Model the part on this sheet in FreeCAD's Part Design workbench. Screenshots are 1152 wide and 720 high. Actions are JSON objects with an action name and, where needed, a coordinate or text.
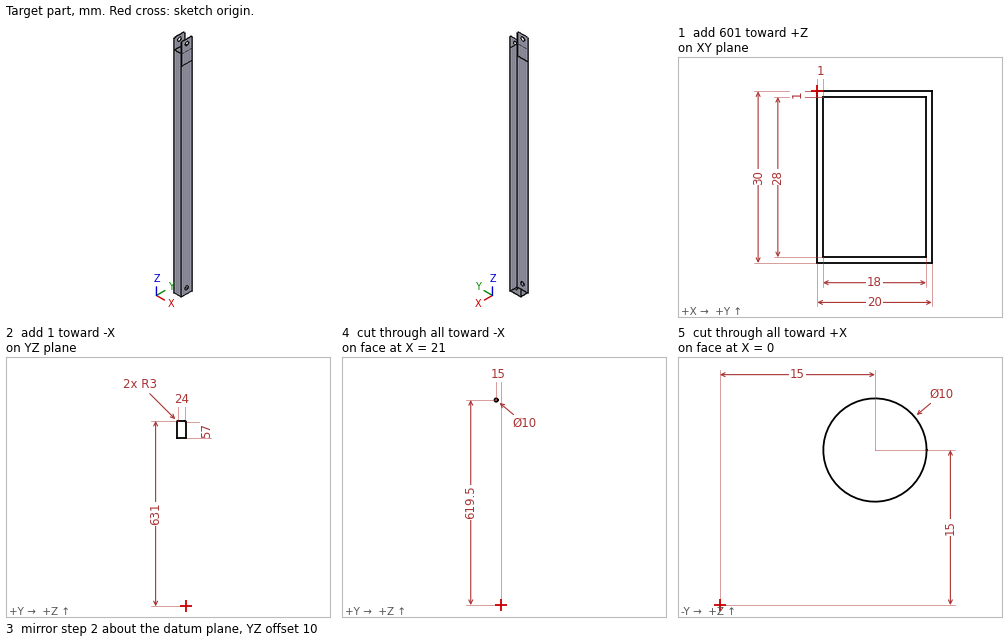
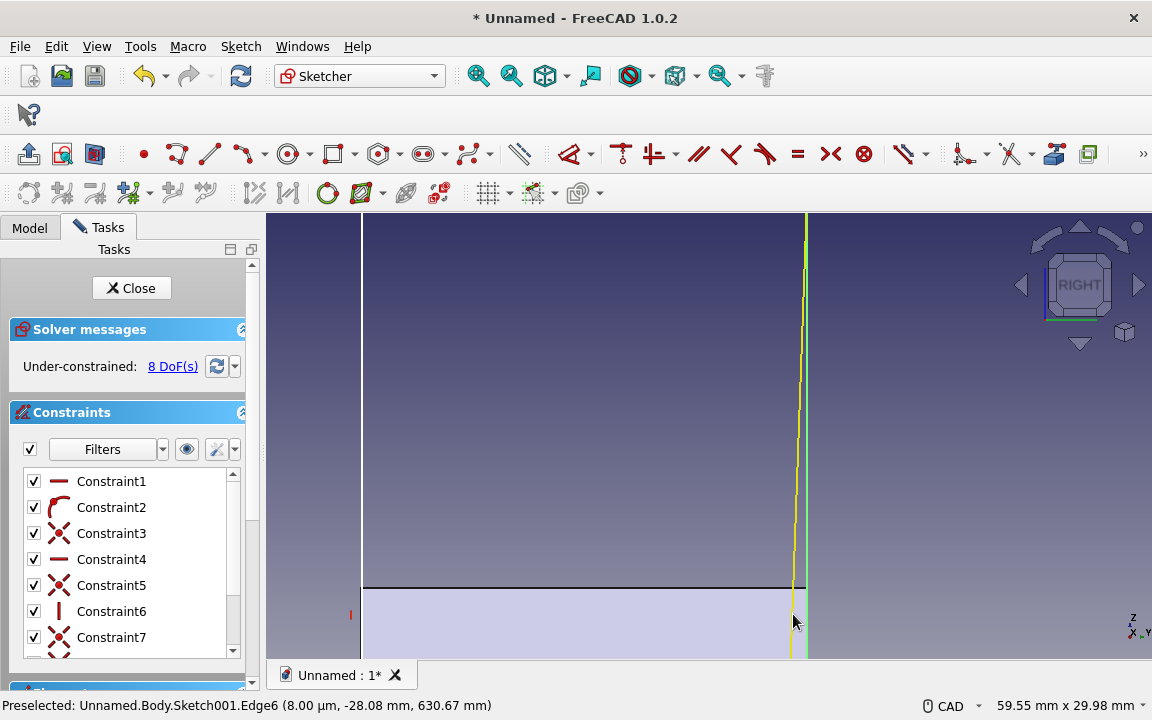
{"action": "left_click", "coordinate": [792, 614]}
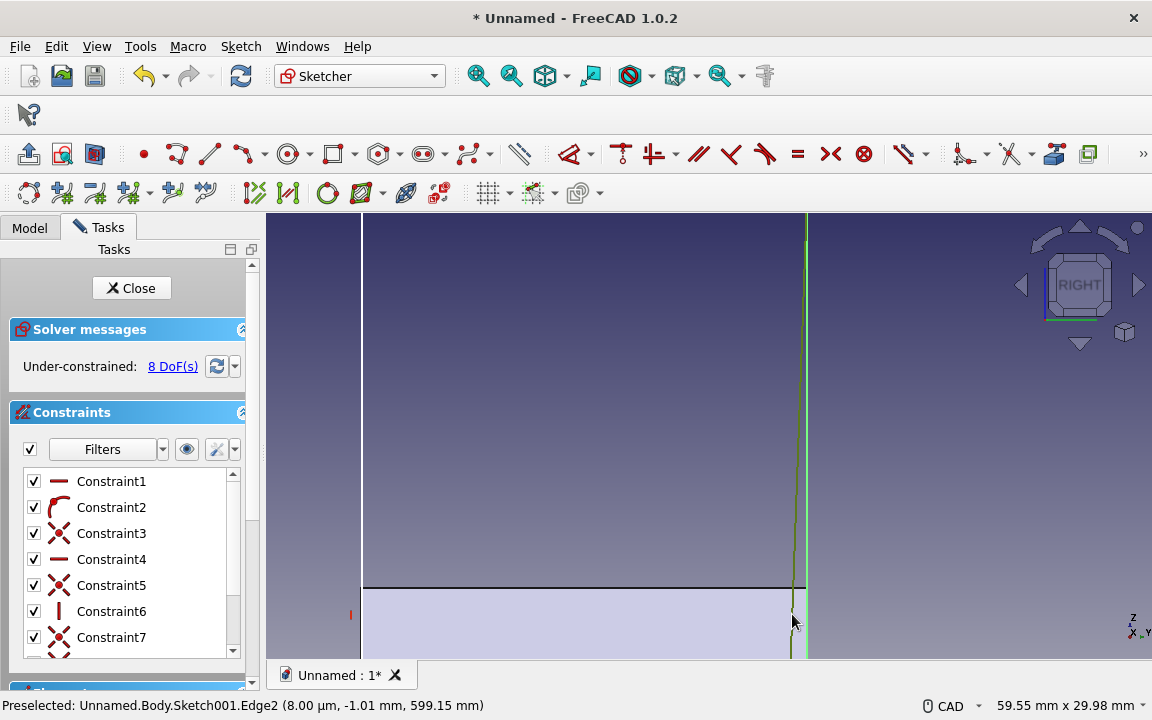
{"action": "scroll", "coordinate": [665, 371], "scroll_direction": "down", "scroll_amount": 6}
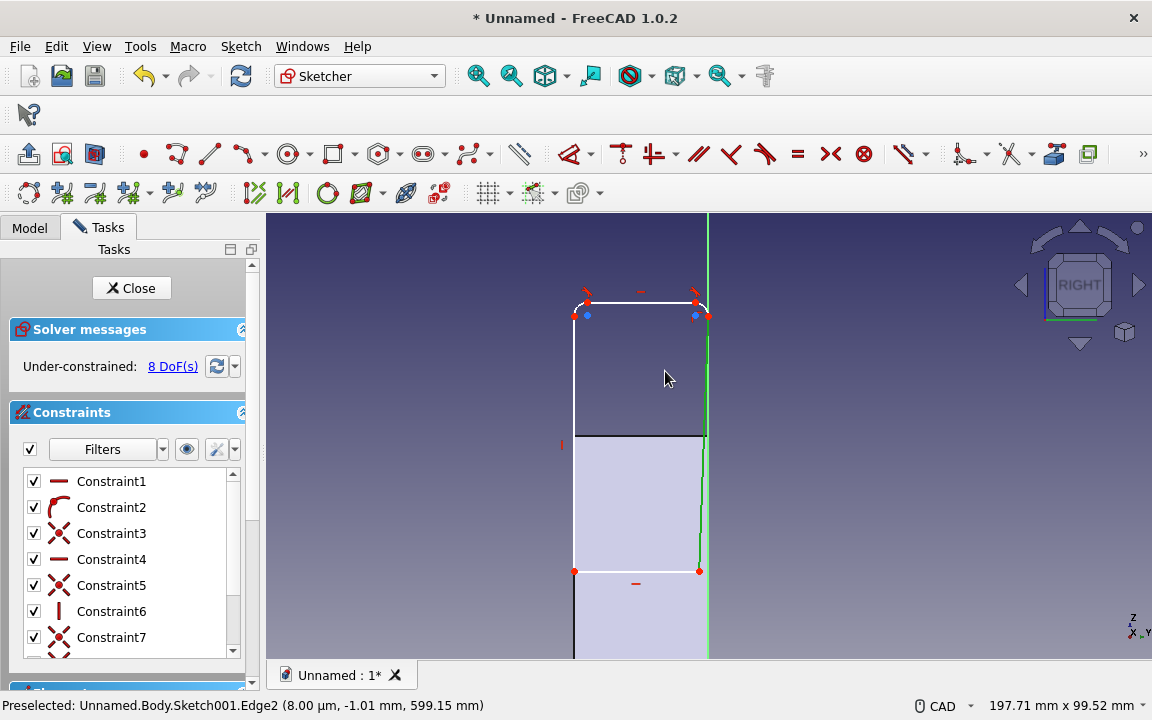
{"action": "scroll", "coordinate": [707, 311], "scroll_direction": "up", "scroll_amount": 4}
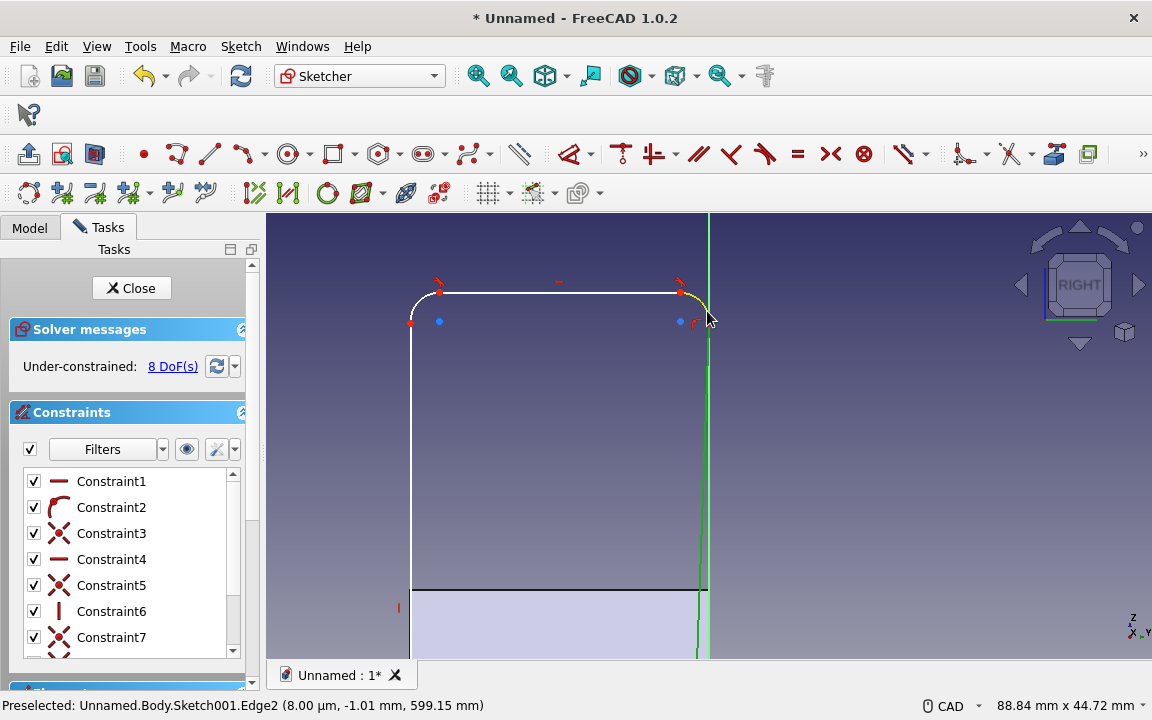
{"action": "left_click", "coordinate": [707, 310]}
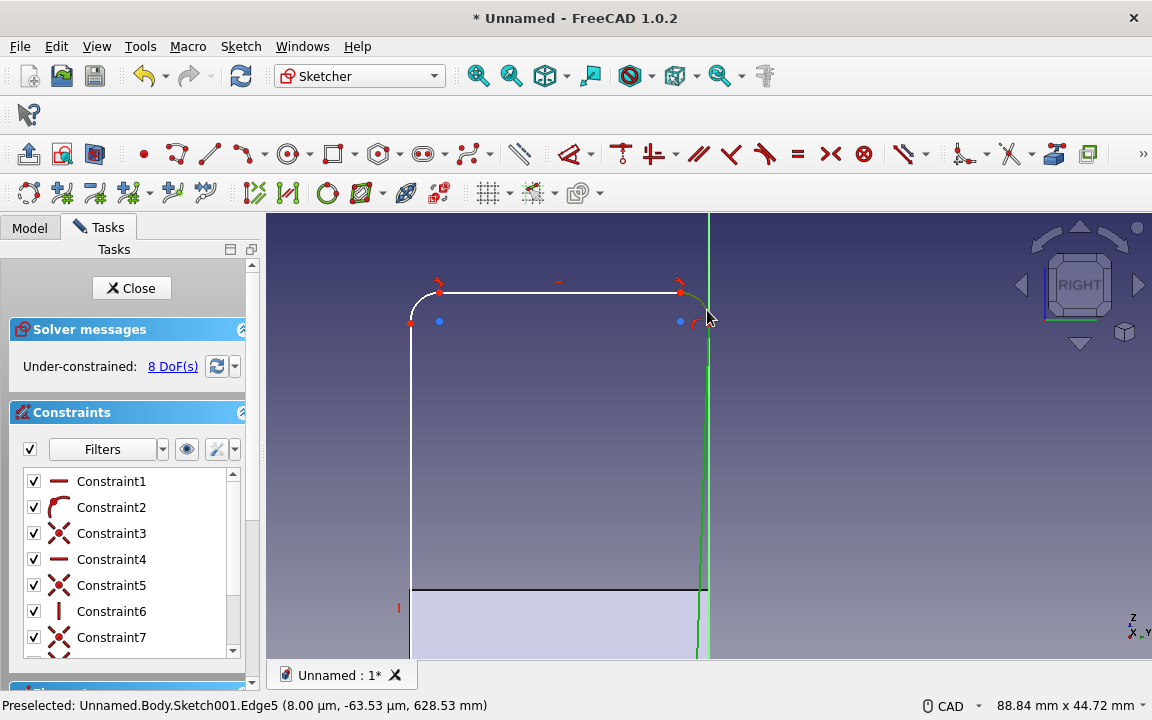
{"action": "key", "text": "t"}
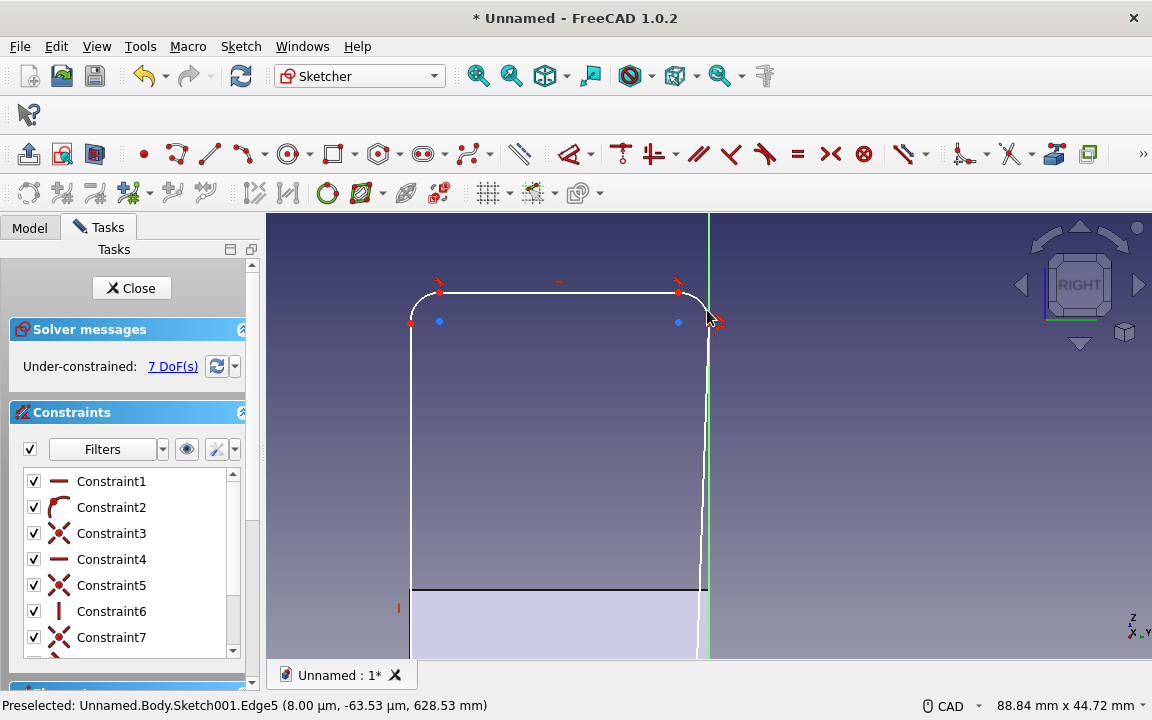
{"action": "left_click", "coordinate": [411, 494]}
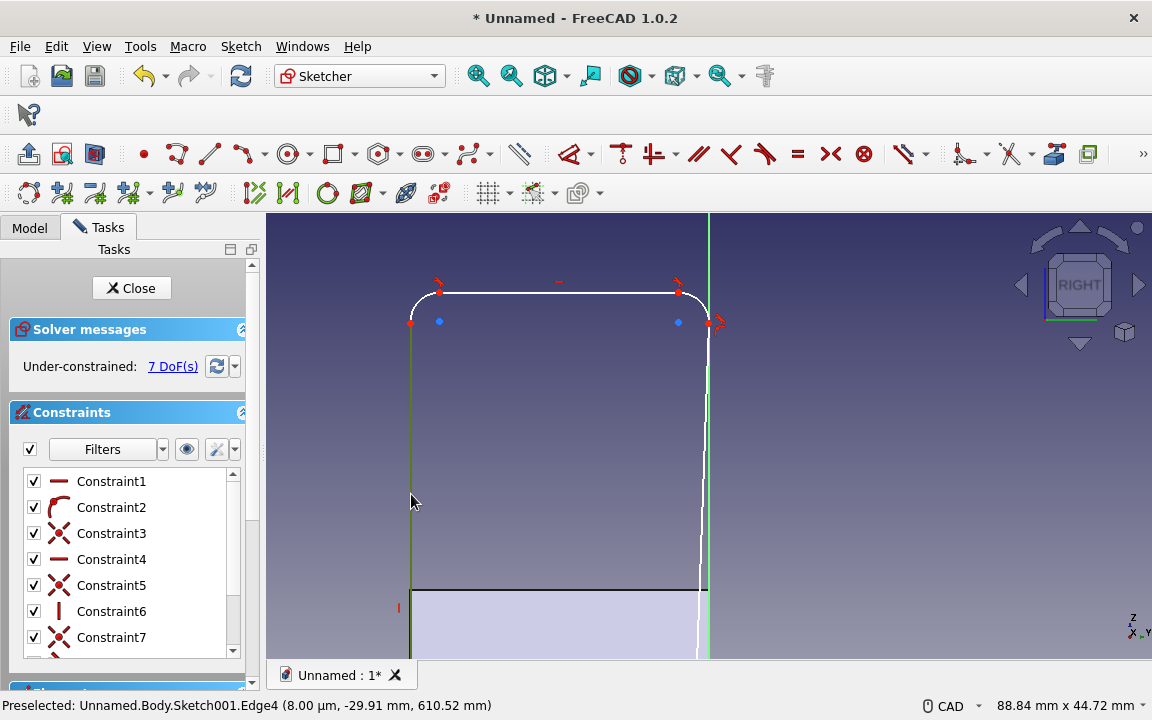
{"action": "left_click", "coordinate": [426, 296]}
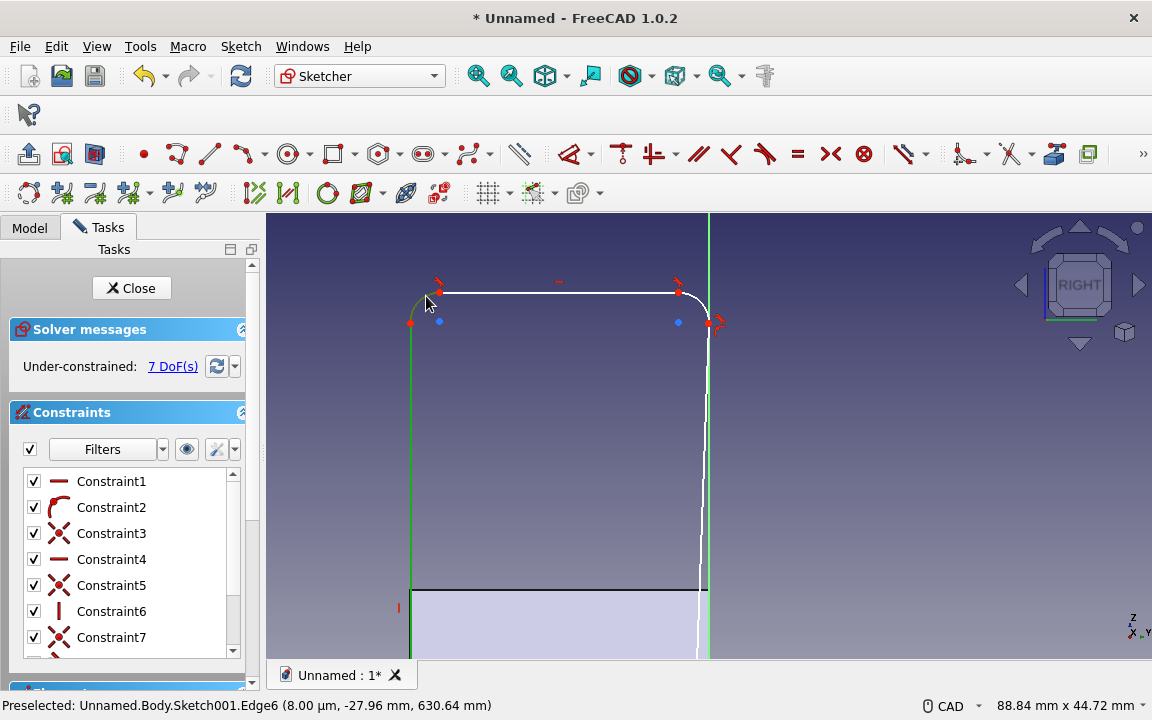
{"action": "key", "text": "t"}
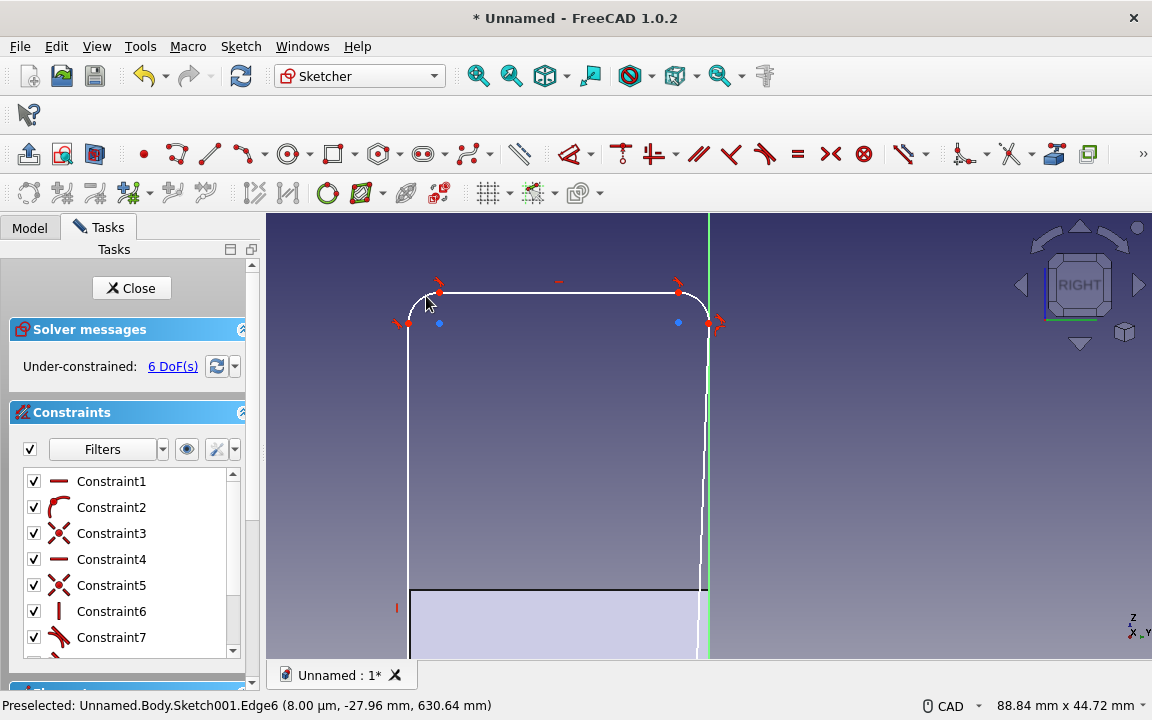
{"action": "scroll", "coordinate": [699, 608], "scroll_direction": "up", "scroll_amount": 2}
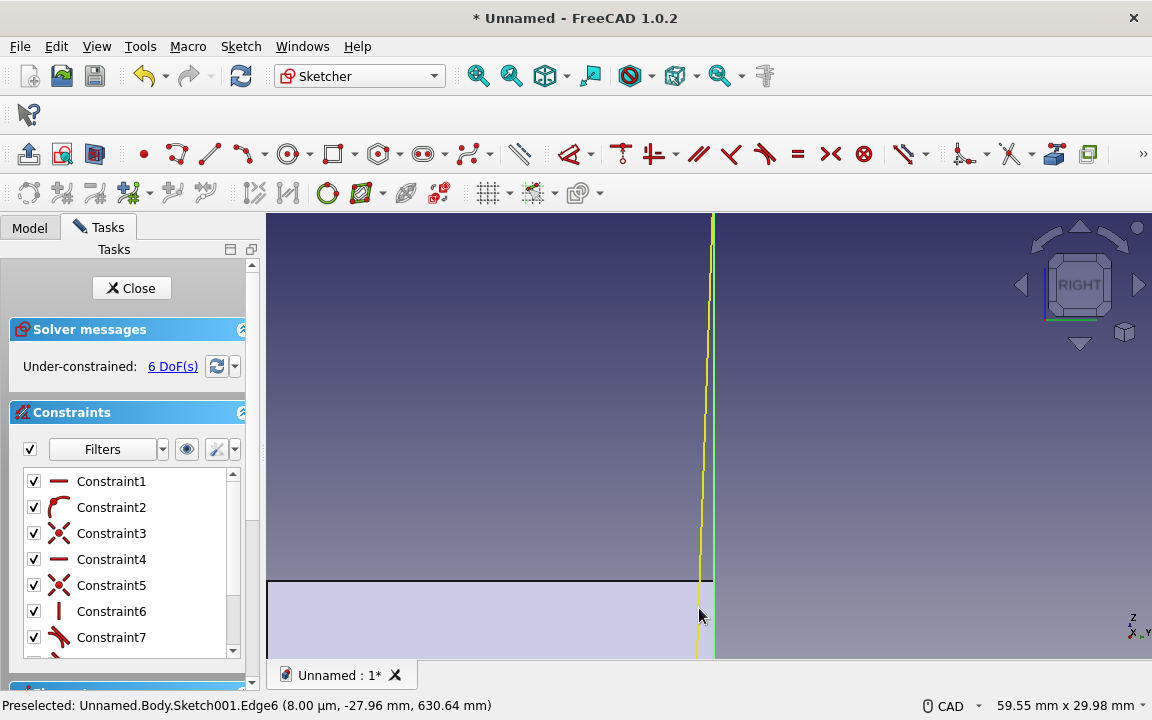
{"action": "left_click", "coordinate": [699, 607]}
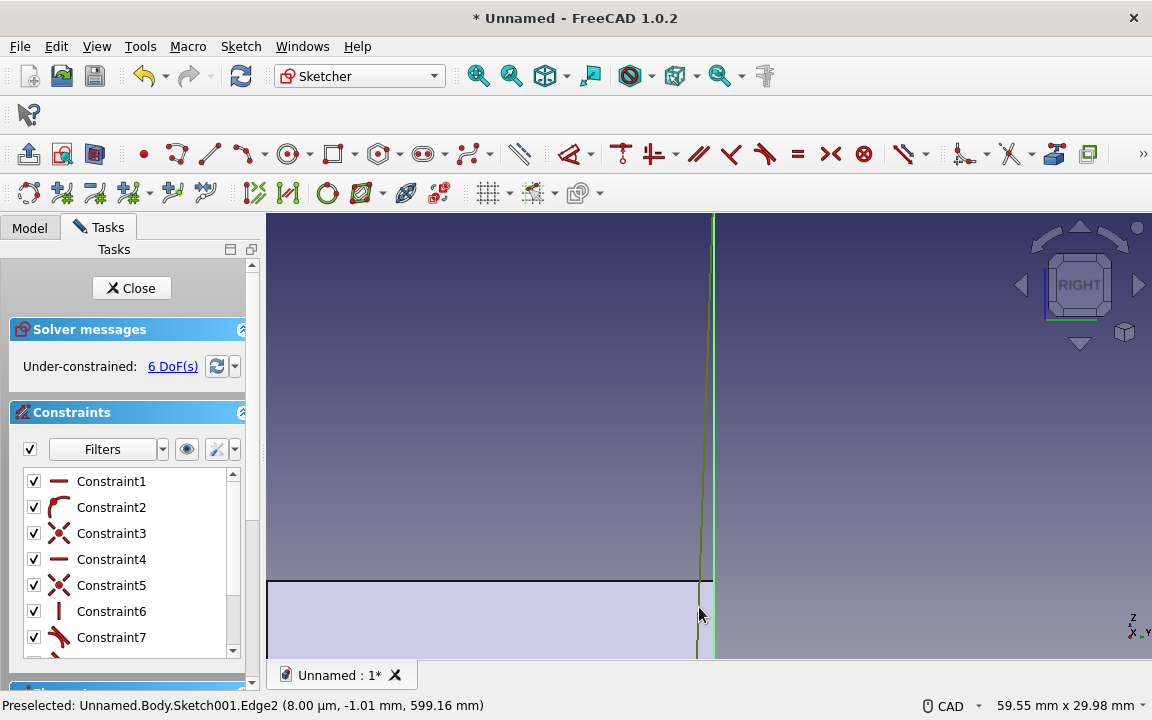
{"action": "key", "text": "v"}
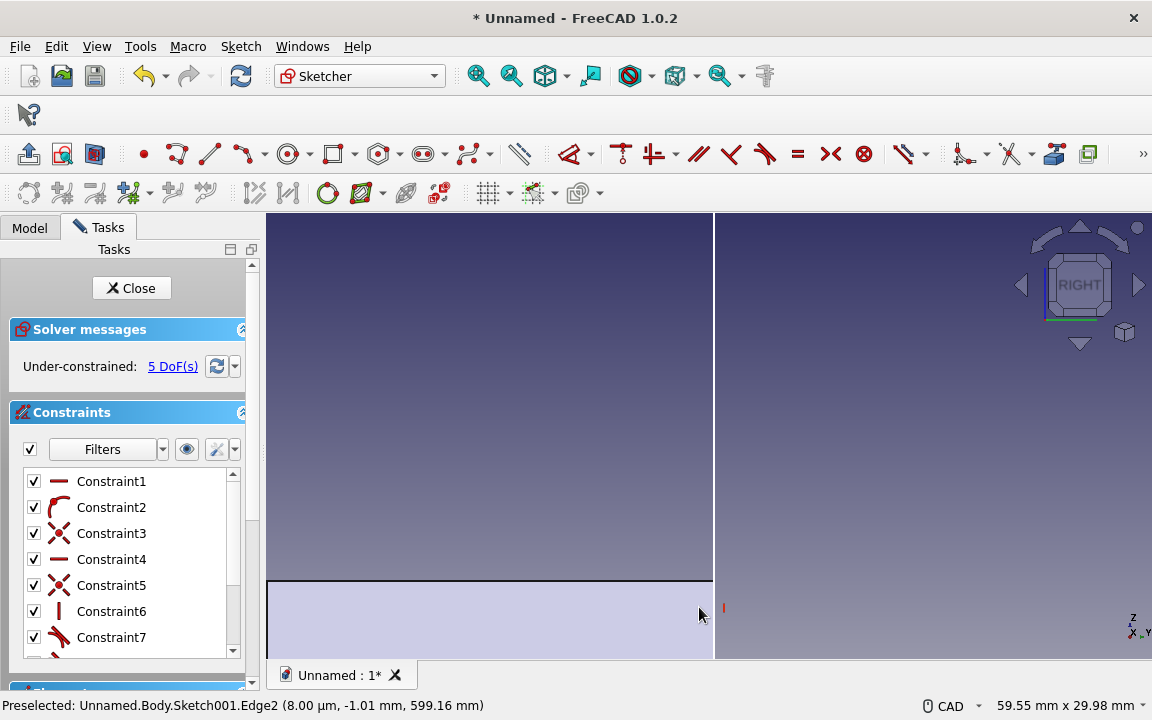
{"action": "scroll", "coordinate": [705, 374], "scroll_direction": "down", "scroll_amount": 6}